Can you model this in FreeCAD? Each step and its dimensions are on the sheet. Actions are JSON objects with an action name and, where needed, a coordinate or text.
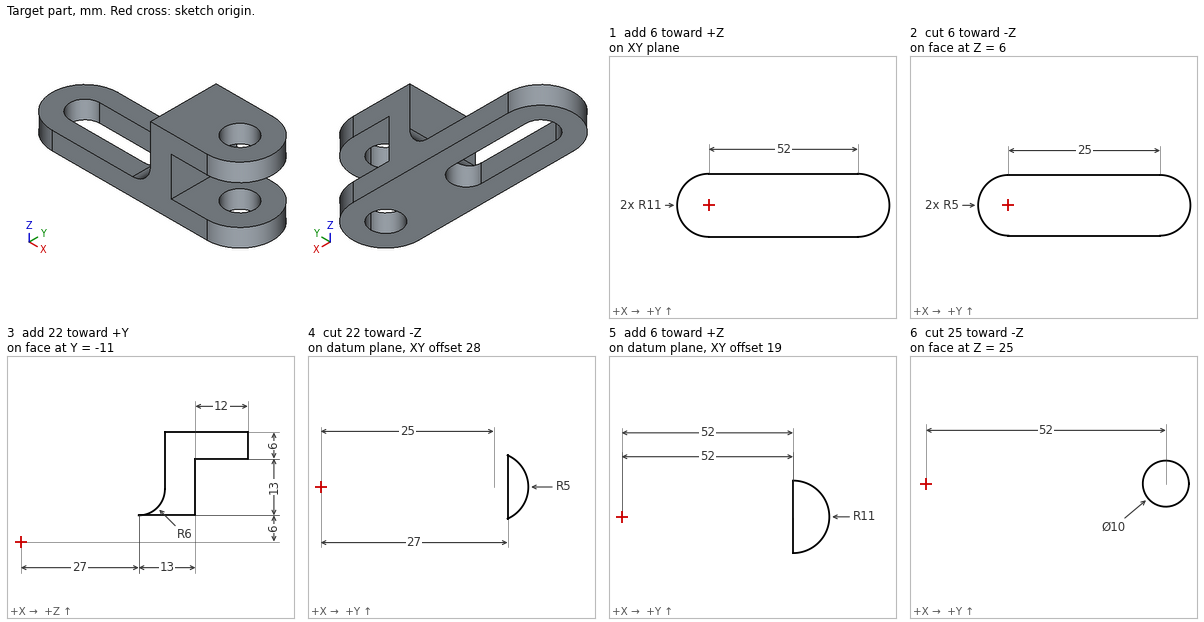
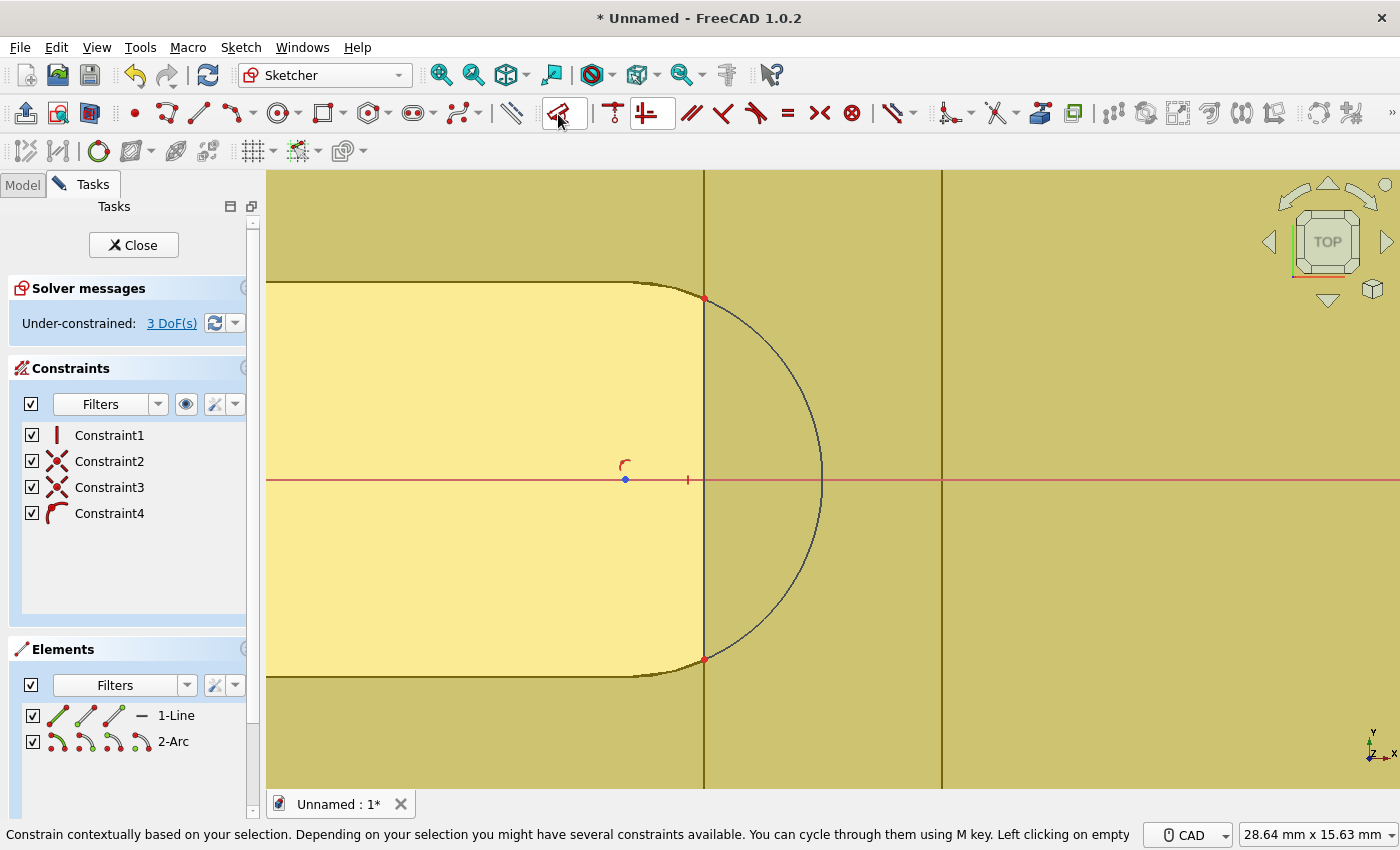
{"action": "left_click", "coordinate": [802, 568]}
{"action": "left_click", "coordinate": [831, 582]}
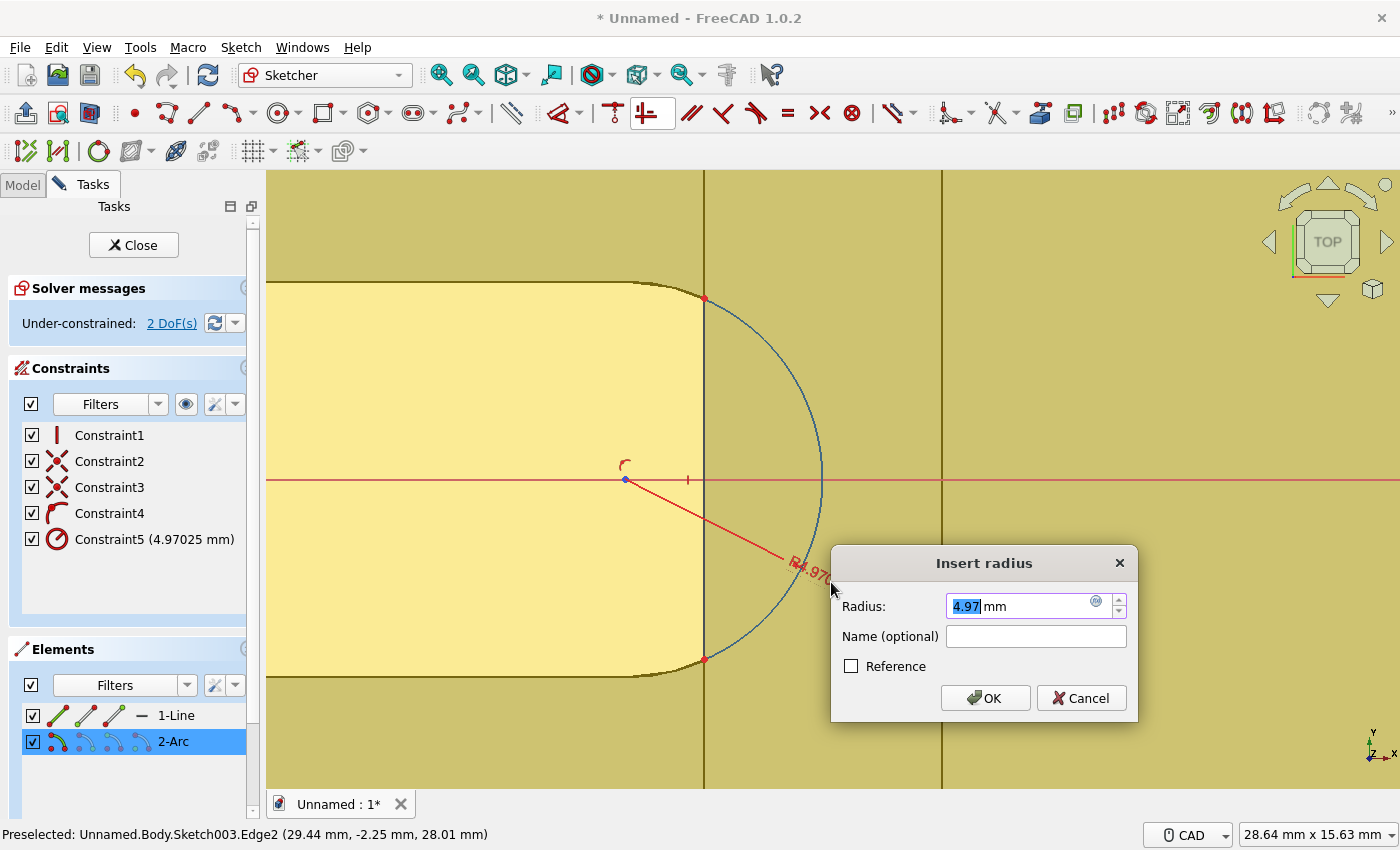
{"action": "type", "text": "5"}
{"action": "key", "text": "Return"}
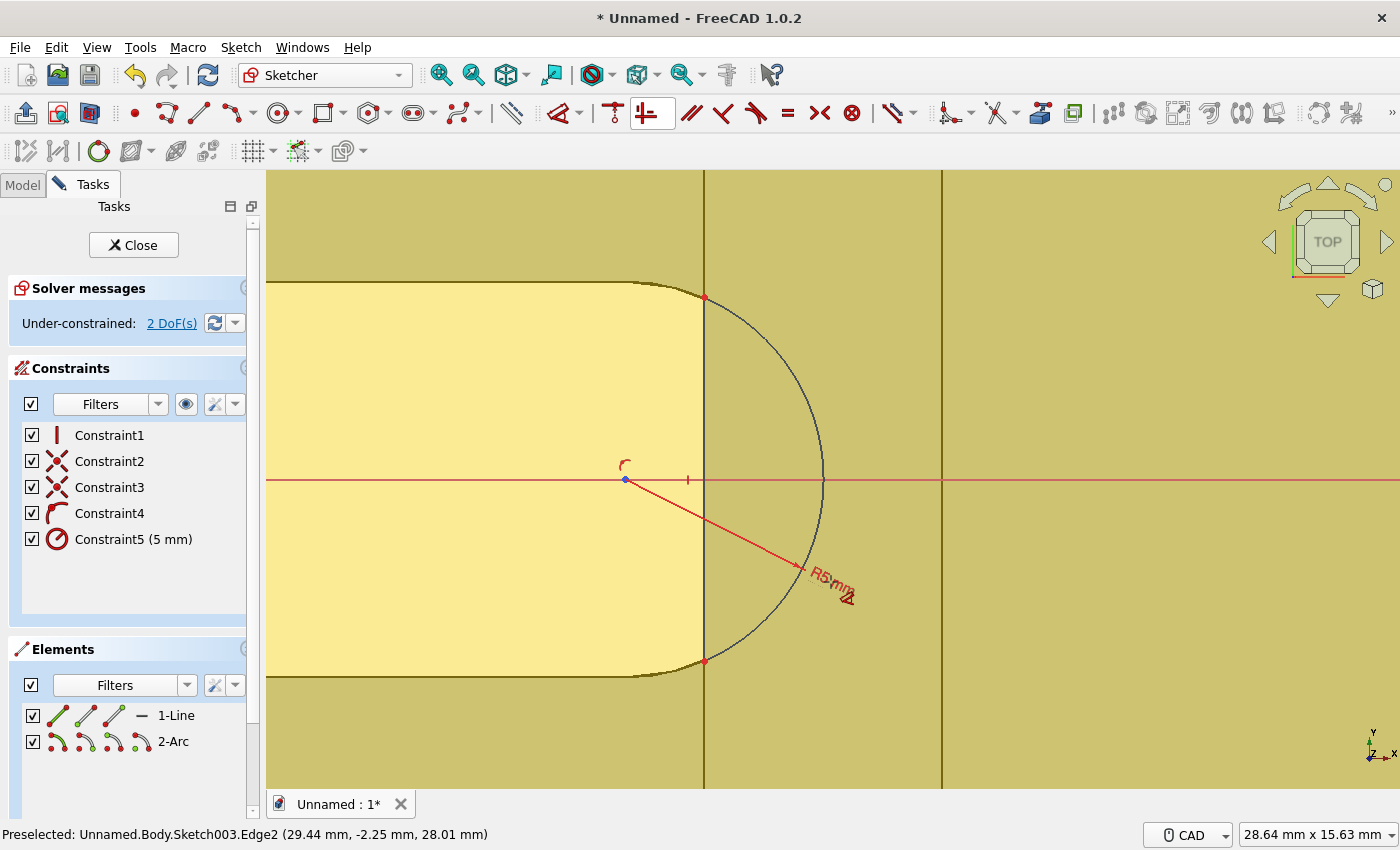
{"action": "left_click", "coordinate": [704, 661]}
{"action": "left_click", "coordinate": [499, 695]}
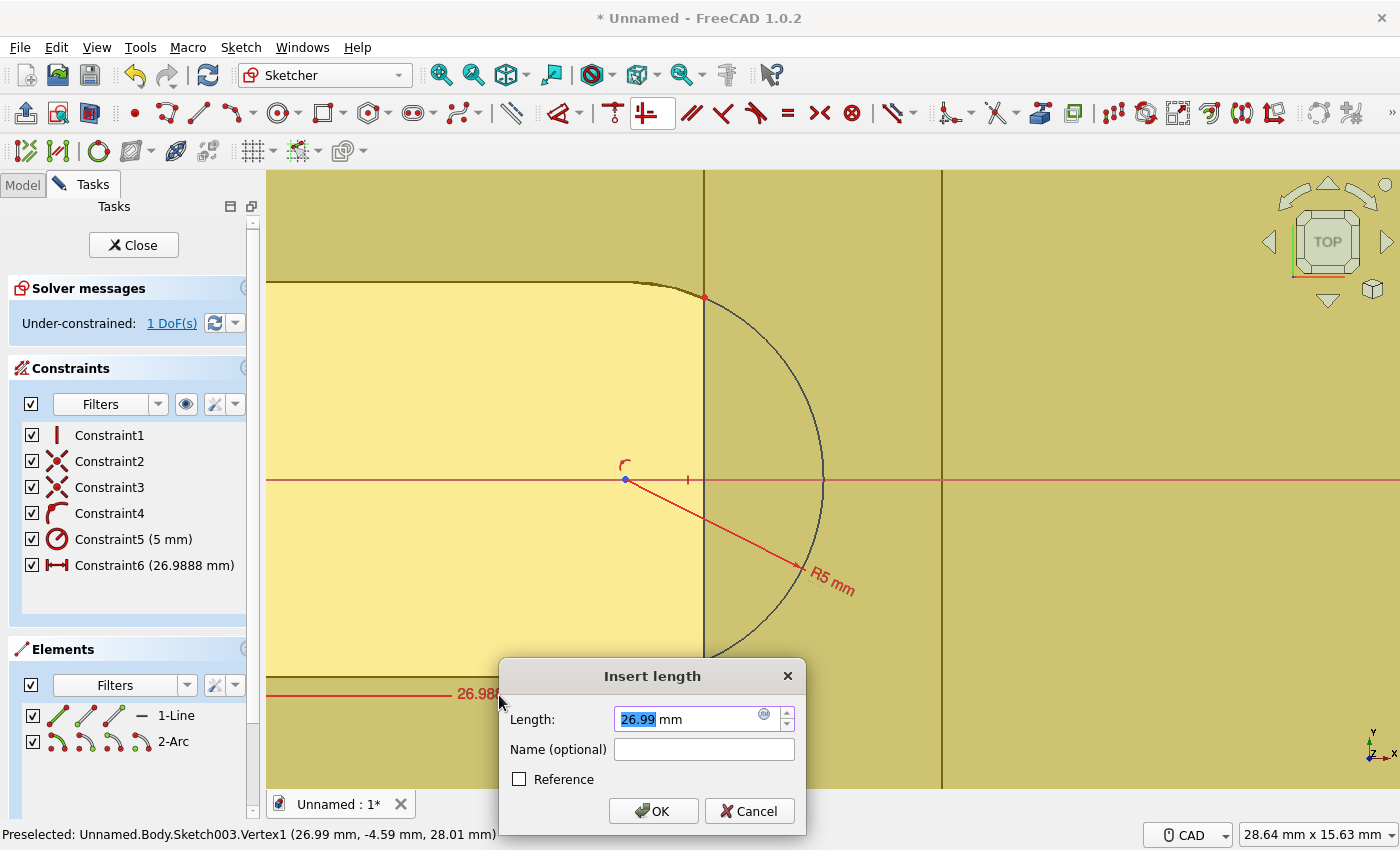
{"action": "type", "text": "27"}
{"action": "key", "text": "Return"}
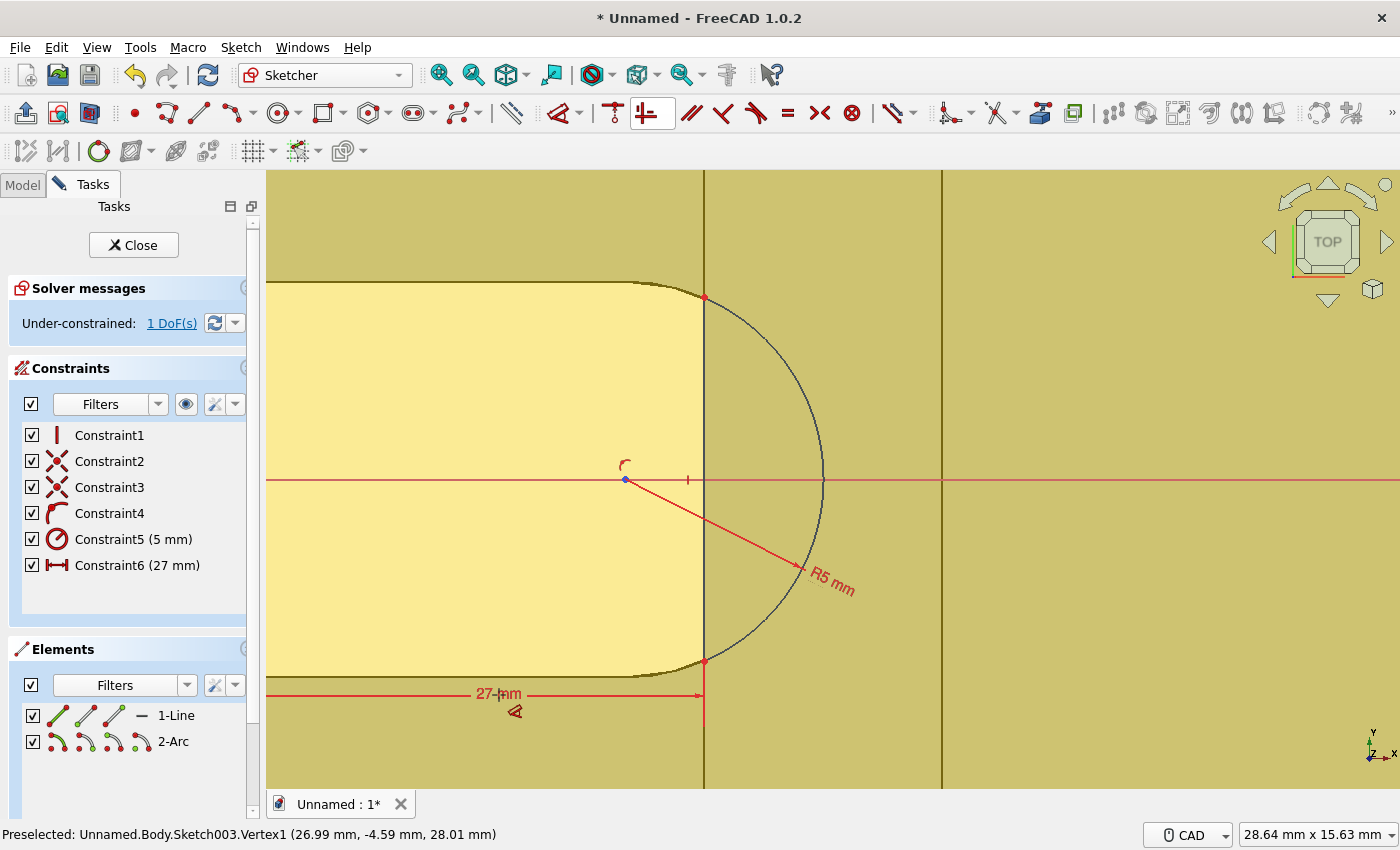
{"action": "left_click", "coordinate": [626, 480]}
{"action": "left_click", "coordinate": [460, 514]}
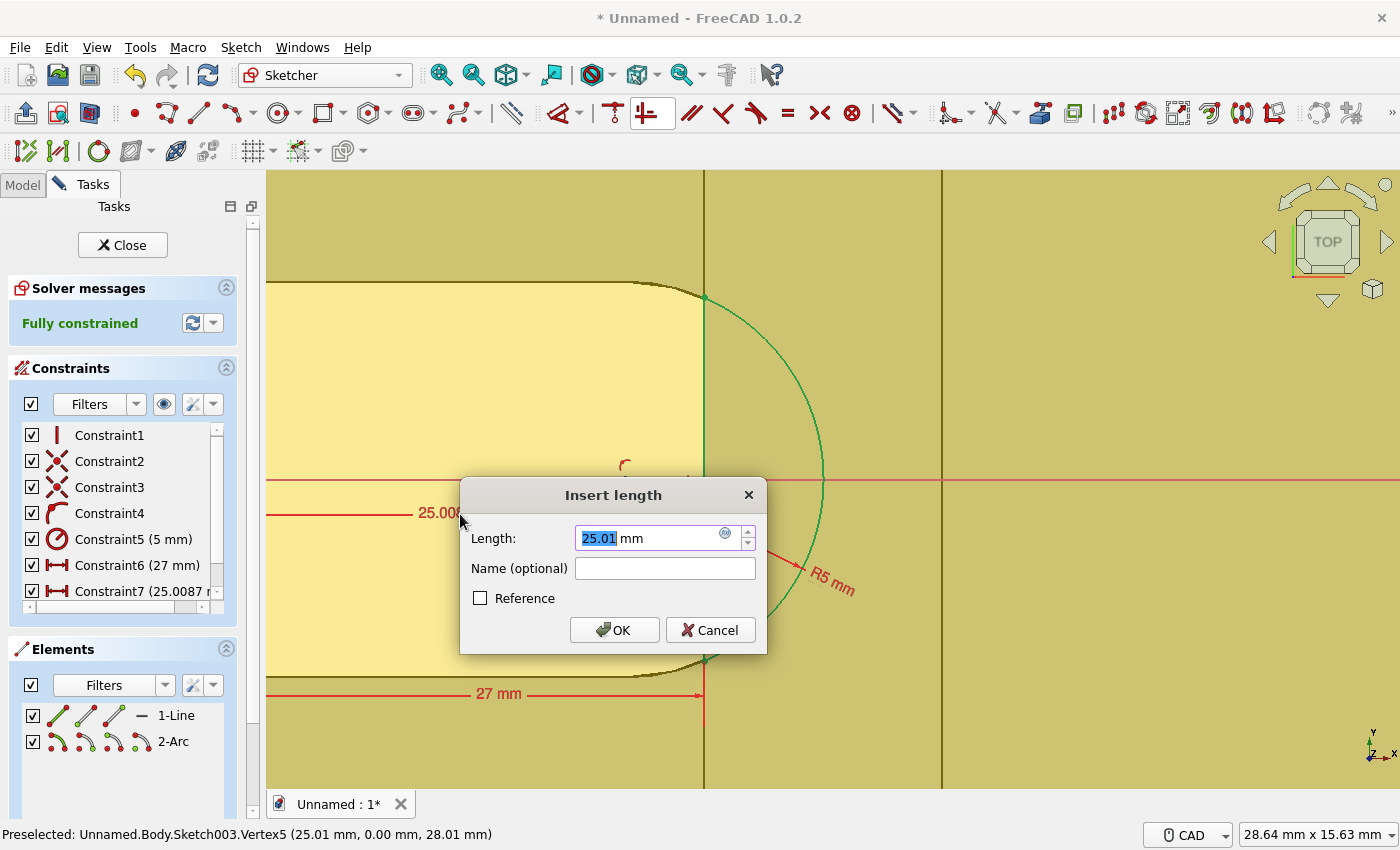
{"action": "type", "text": "25"}
{"action": "key", "text": "Return"}
{"action": "key", "text": "Escape"}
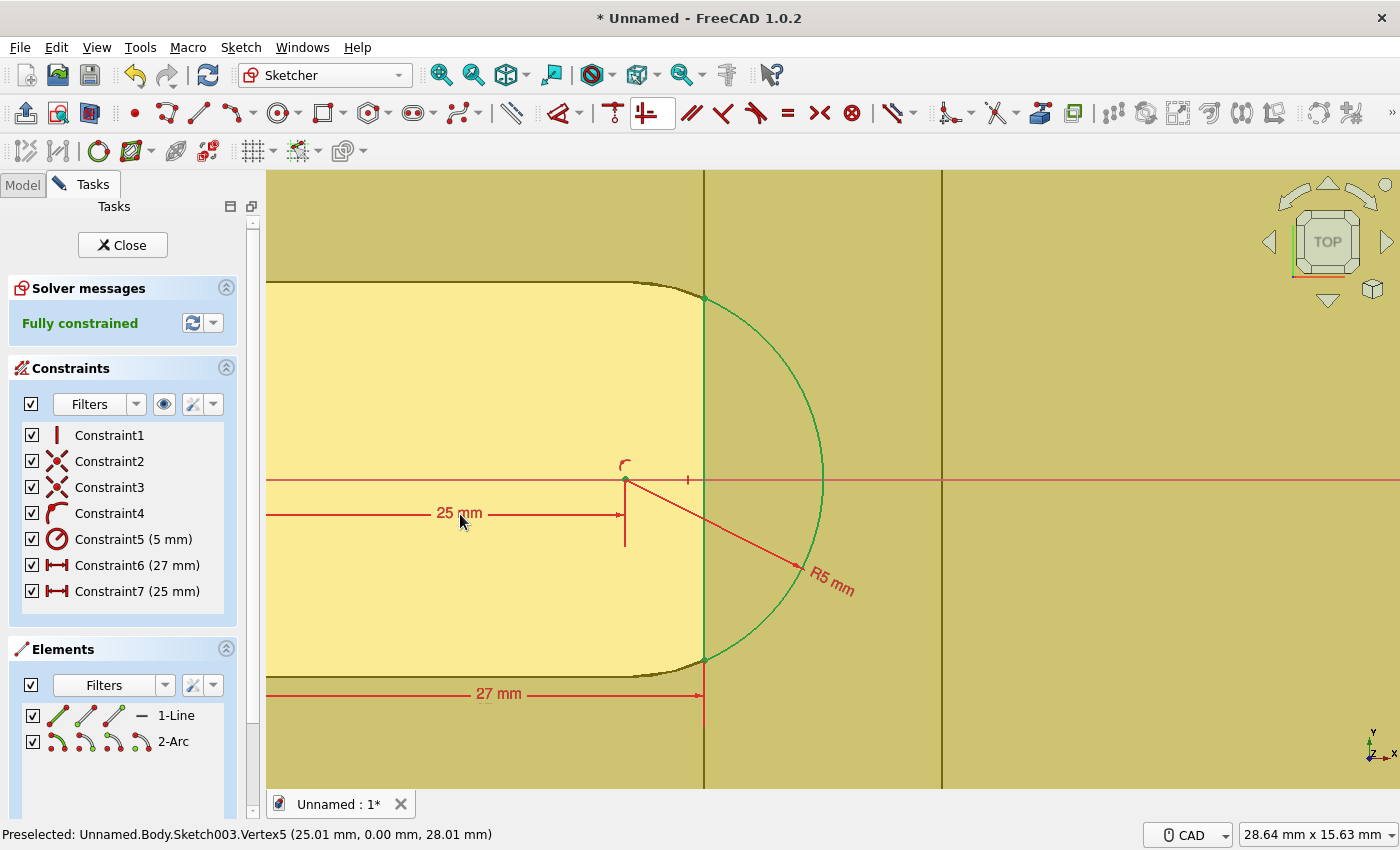
{"action": "left_click", "coordinate": [123, 245]}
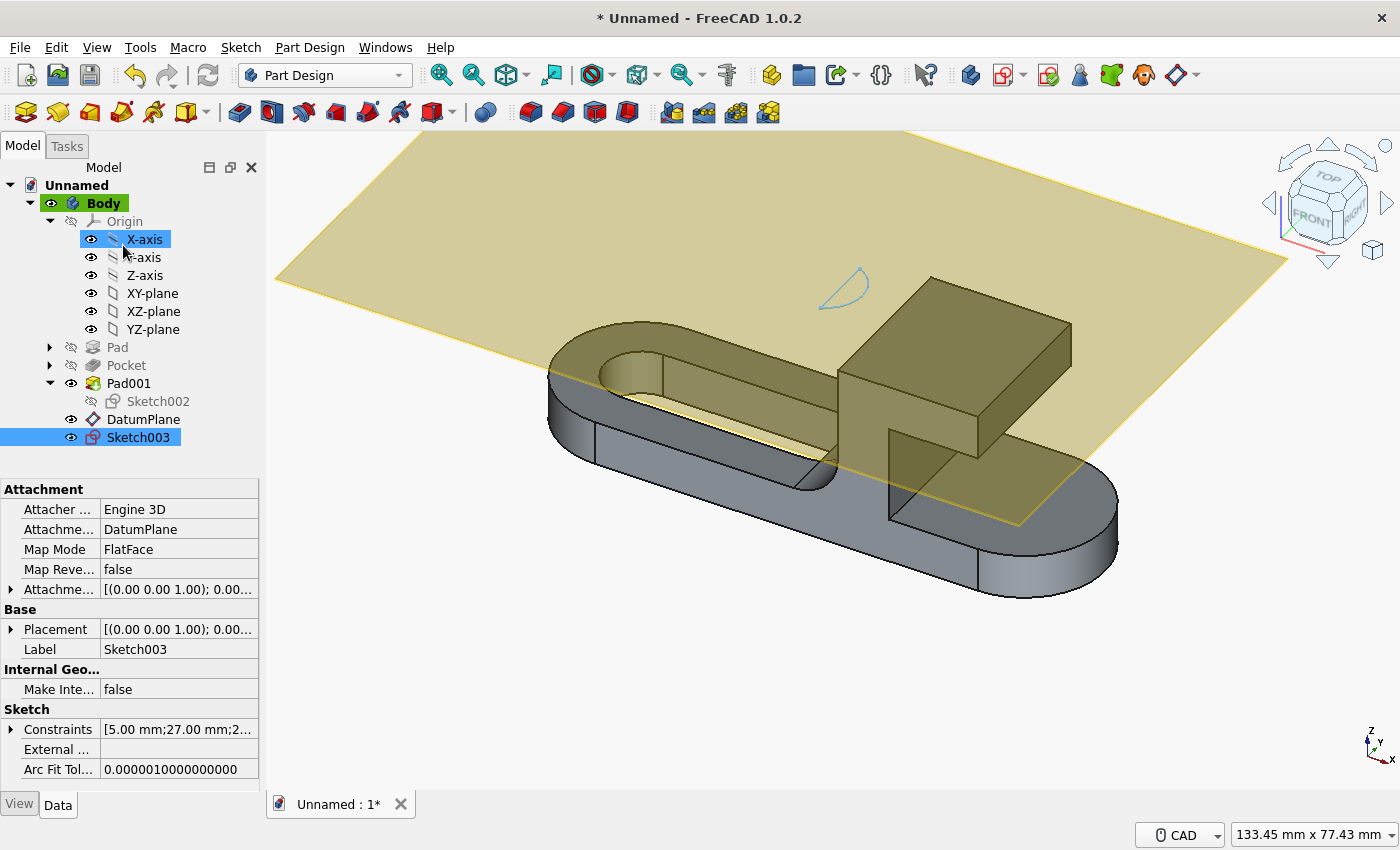
{"action": "left_click", "coordinate": [240, 112]}